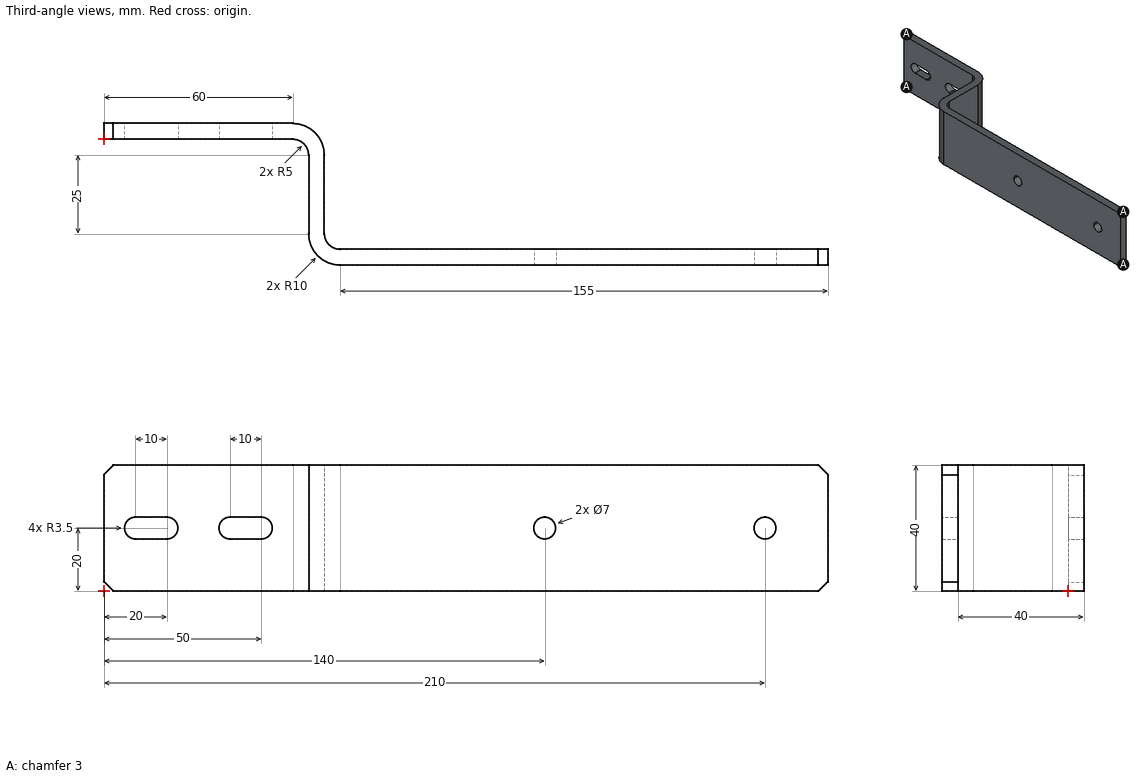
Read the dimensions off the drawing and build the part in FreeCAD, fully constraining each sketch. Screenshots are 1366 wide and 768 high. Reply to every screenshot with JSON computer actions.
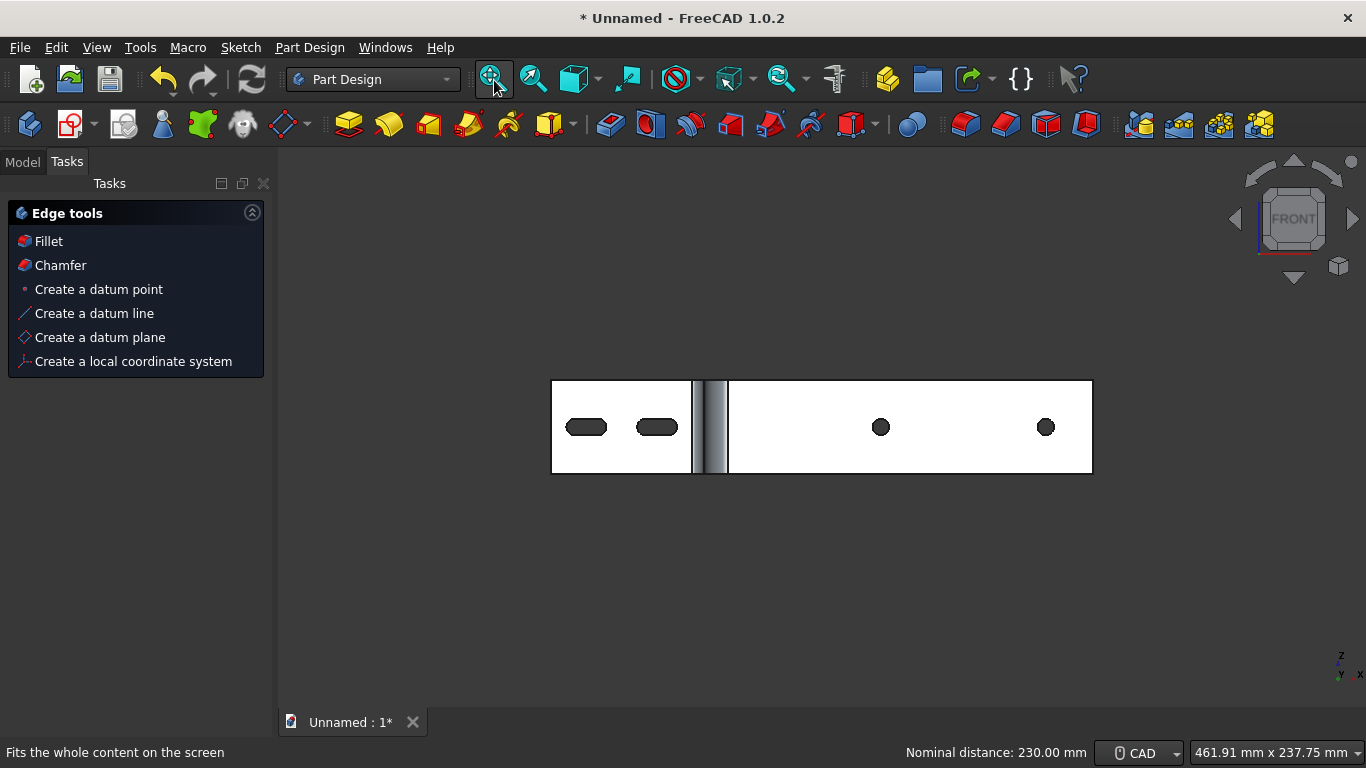
{"action": "key", "text": "3"}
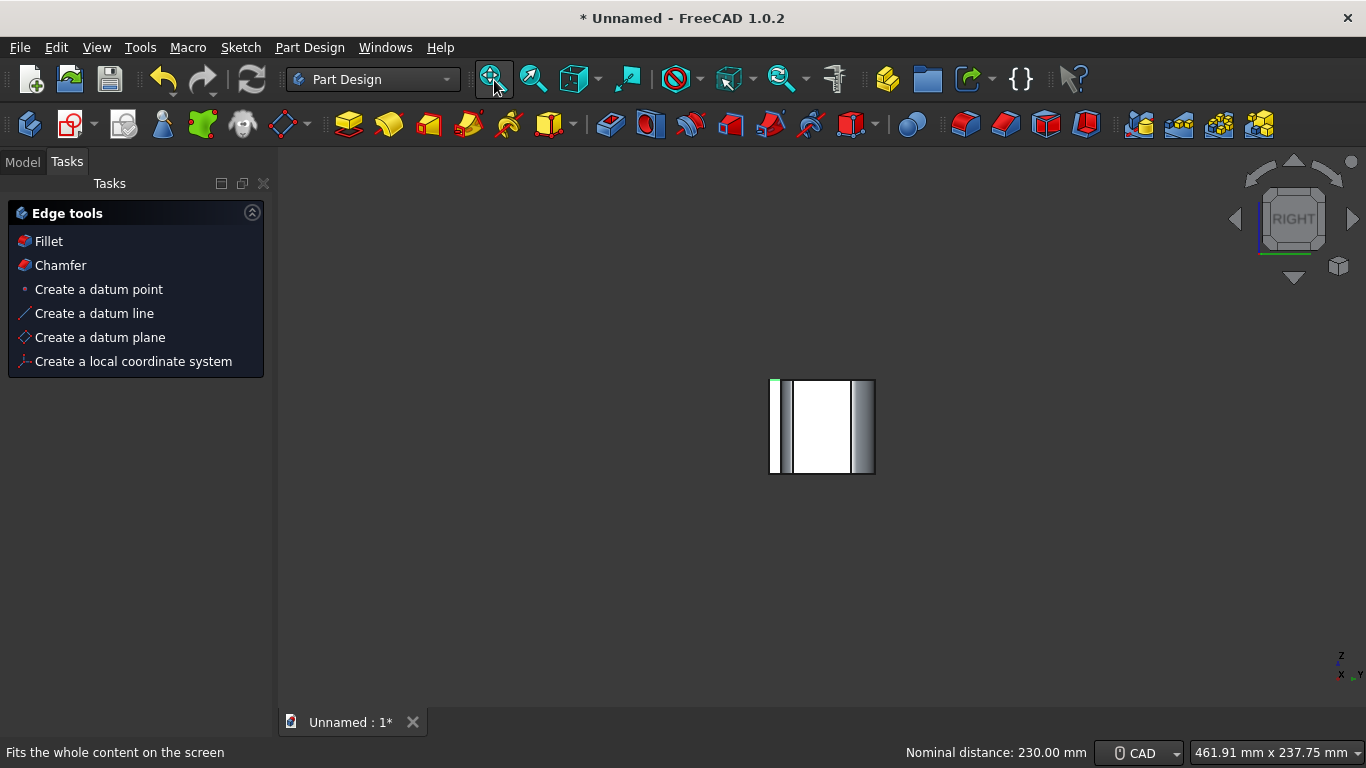
{"action": "left_click", "coordinate": [494, 80]}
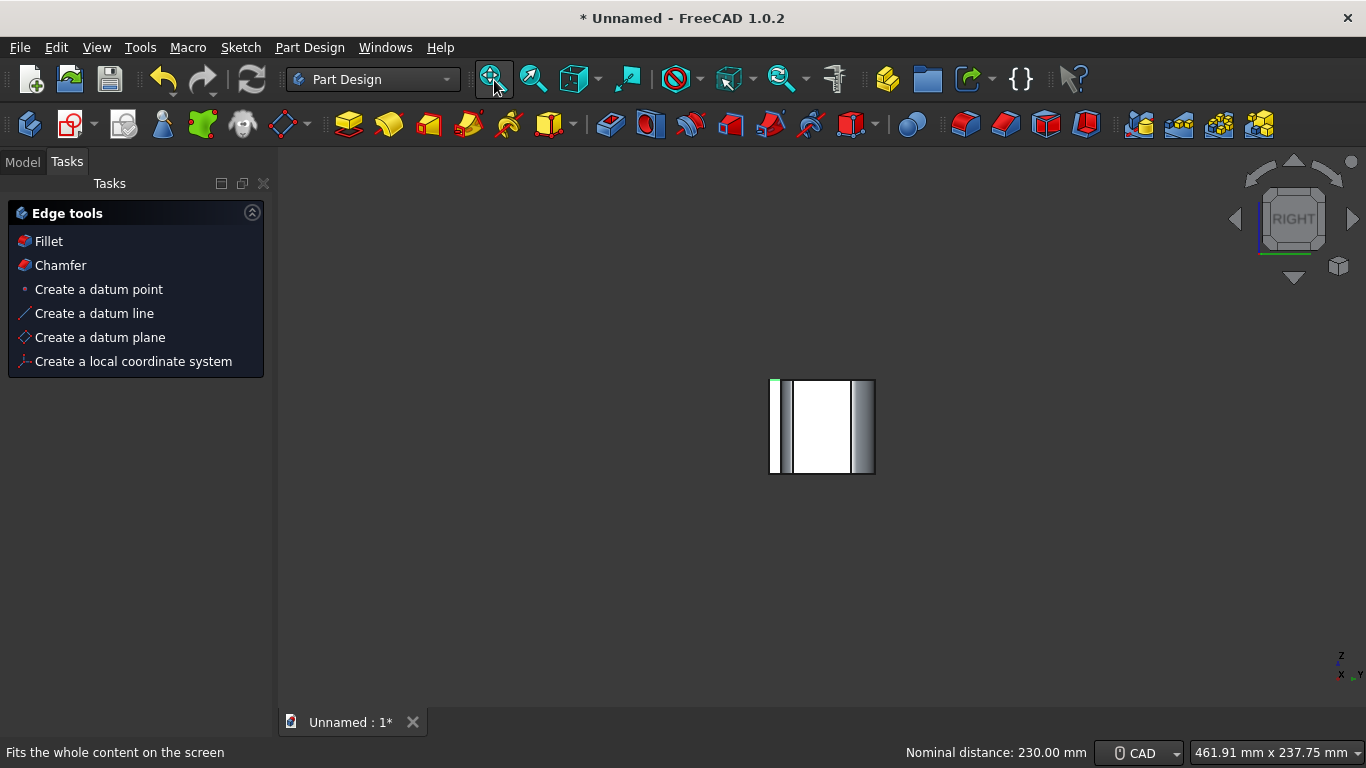
{"action": "scroll", "coordinate": [869, 473], "scroll_direction": "up", "scroll_amount": 7}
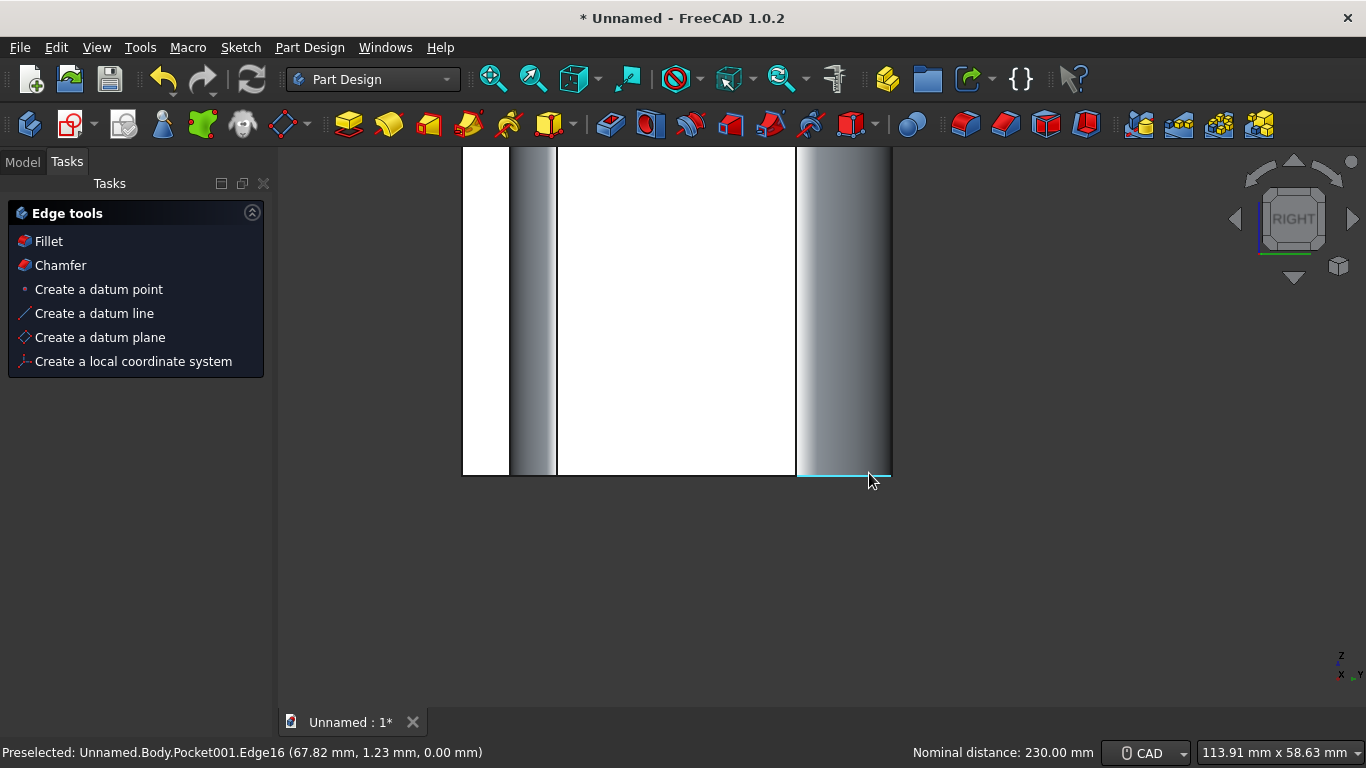
{"action": "left_click", "coordinate": [486, 475], "text": "ctrl"}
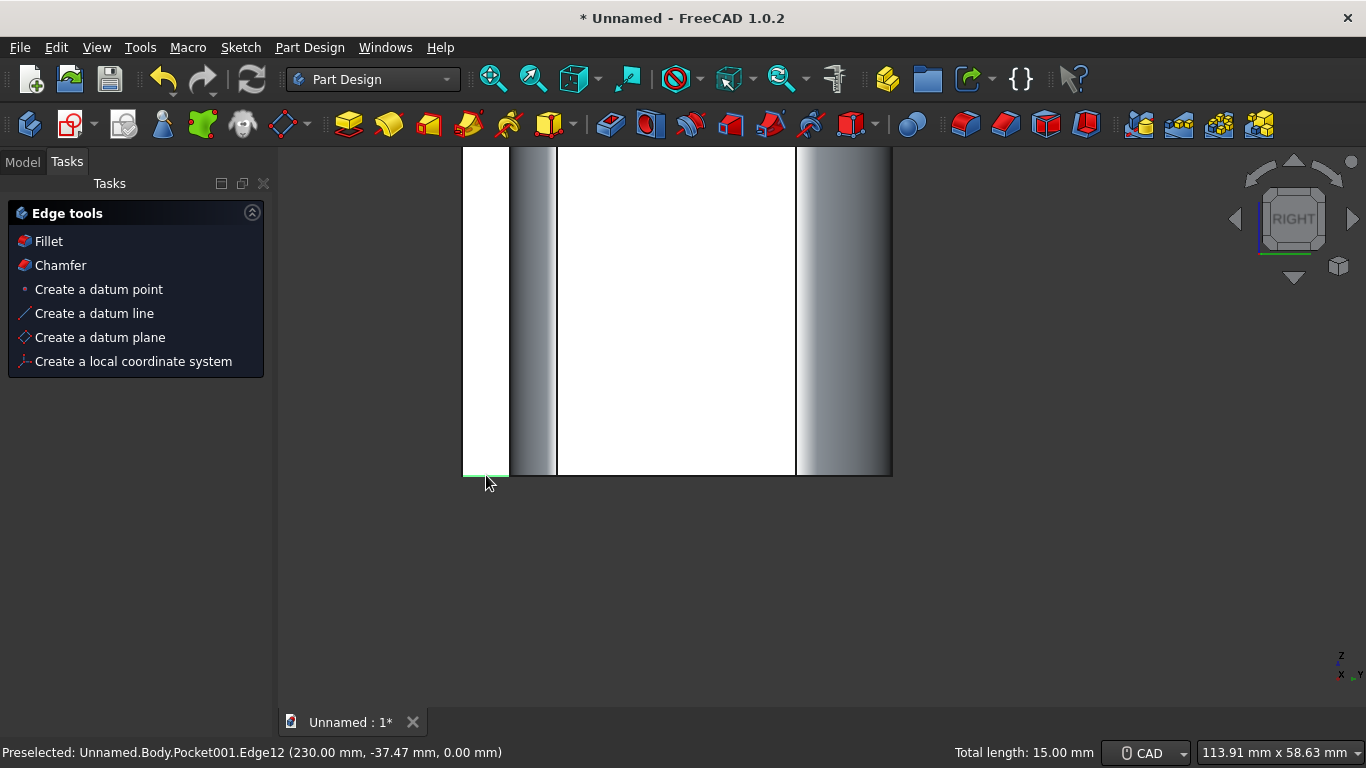
{"action": "left_click", "coordinate": [494, 80]}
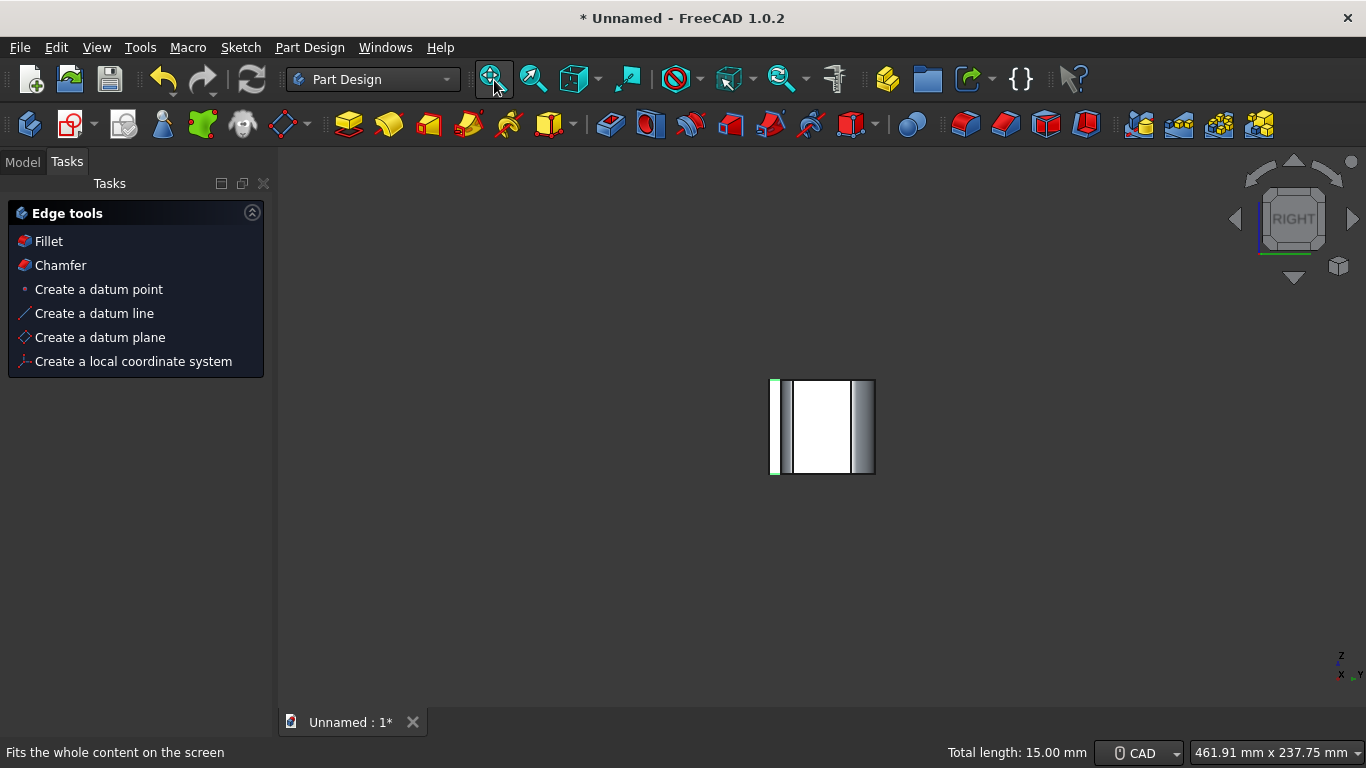
{"action": "key", "text": "5"}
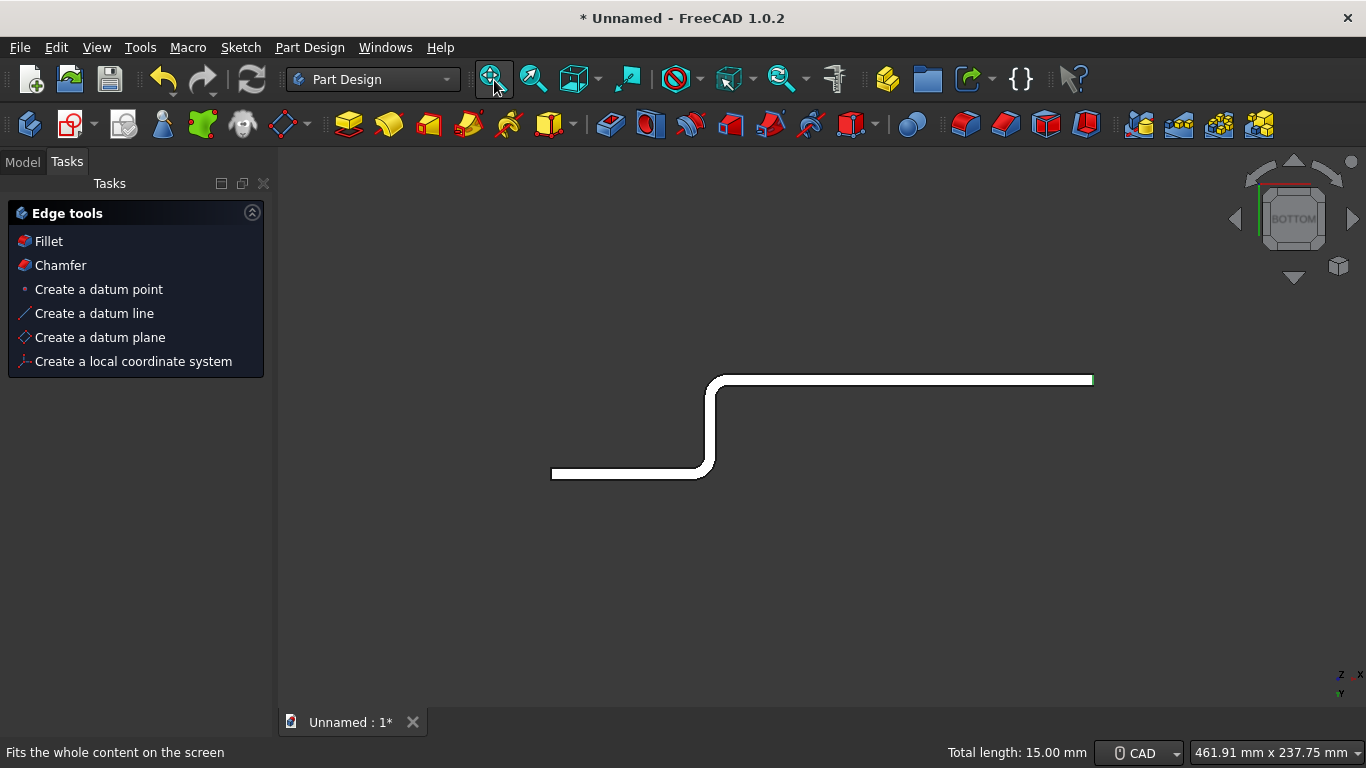
{"action": "scroll", "coordinate": [551, 473], "scroll_direction": "up", "scroll_amount": 7}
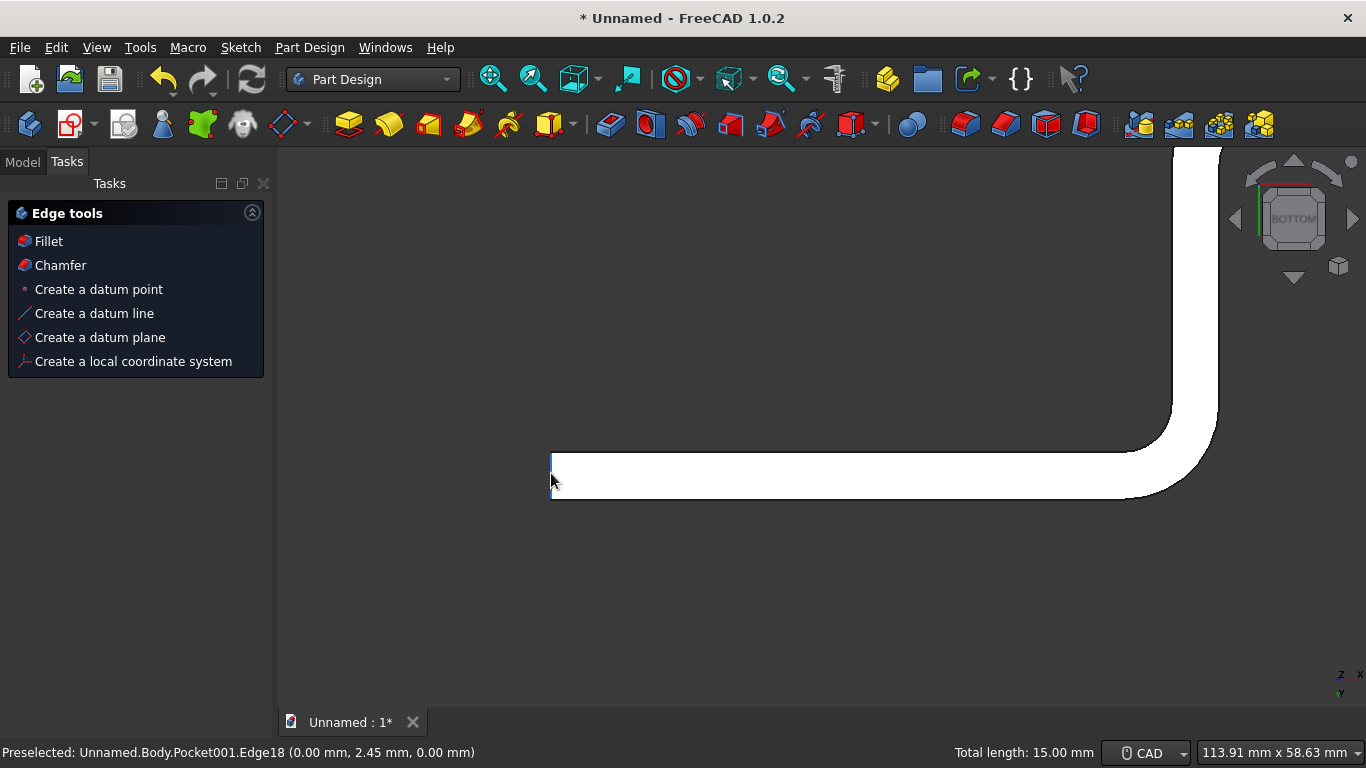
{"action": "left_click", "coordinate": [551, 475], "text": "ctrl"}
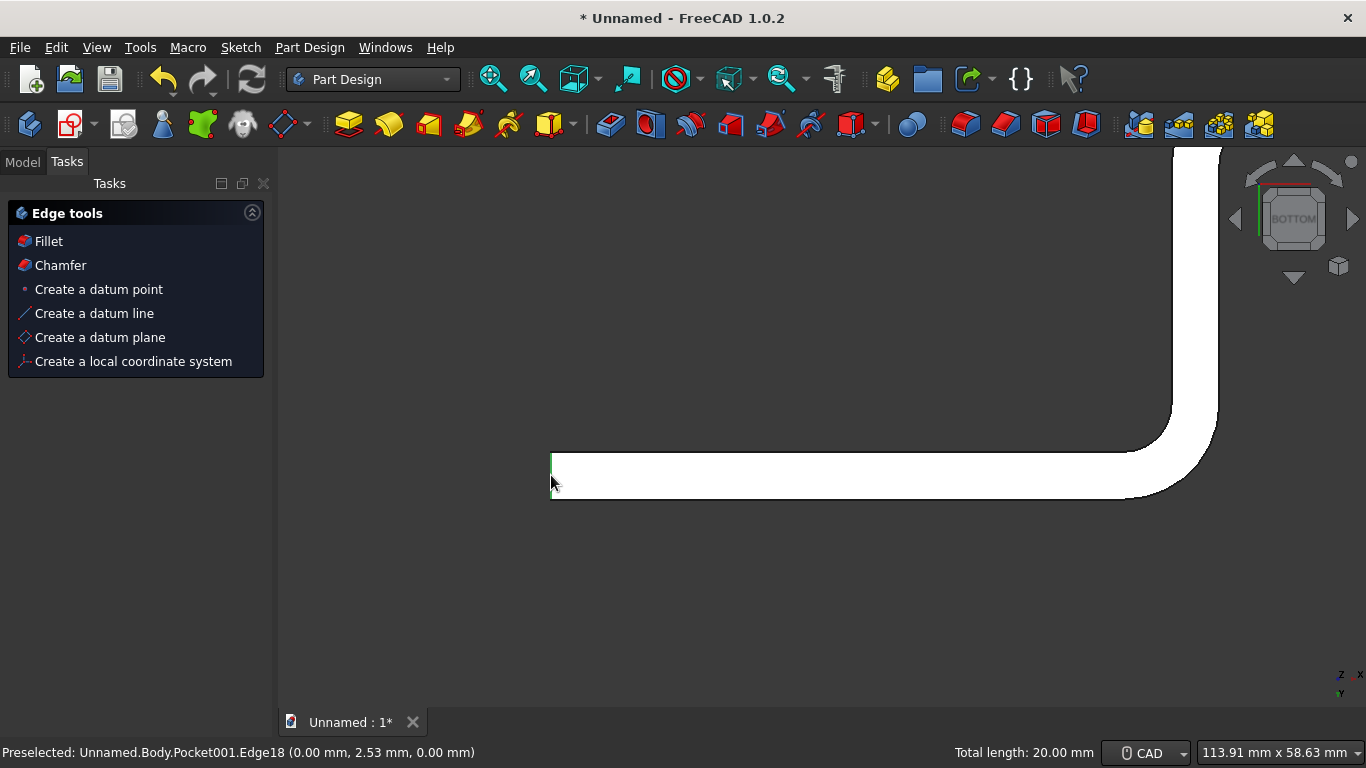
{"action": "left_click", "coordinate": [1006, 124]}